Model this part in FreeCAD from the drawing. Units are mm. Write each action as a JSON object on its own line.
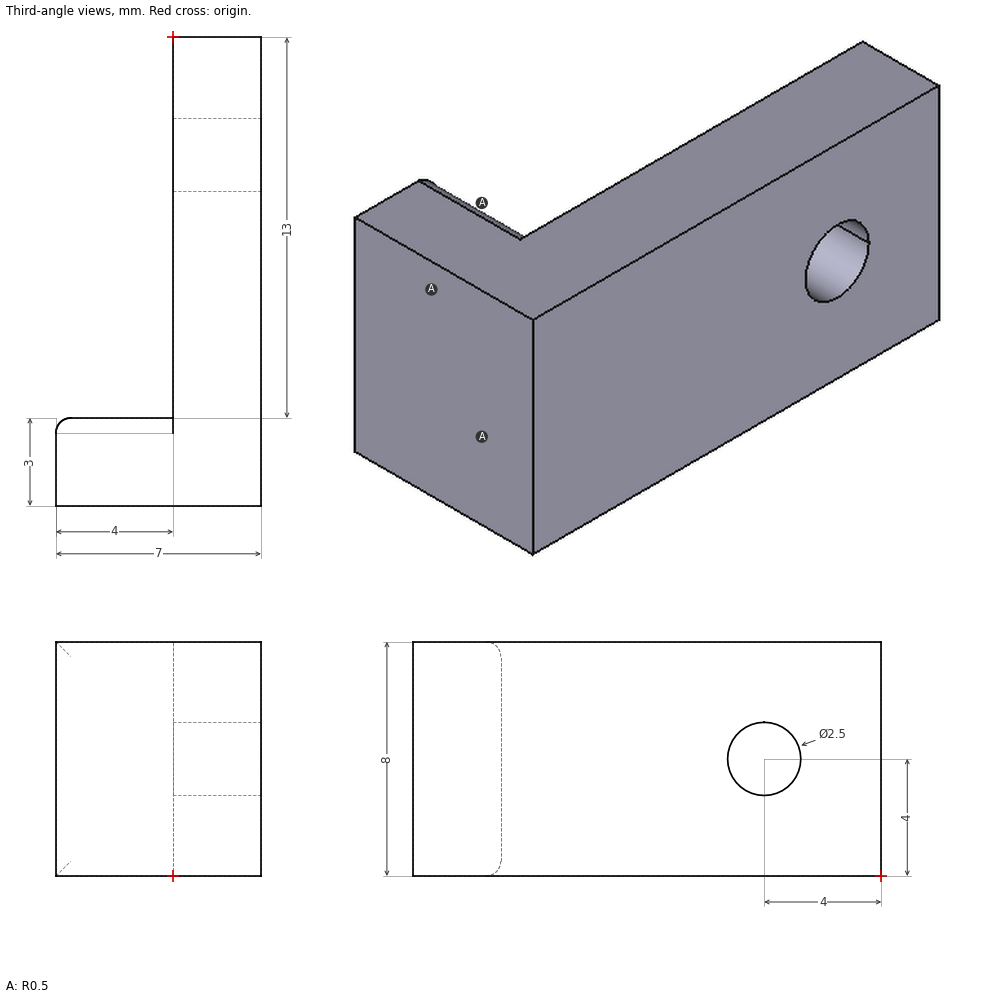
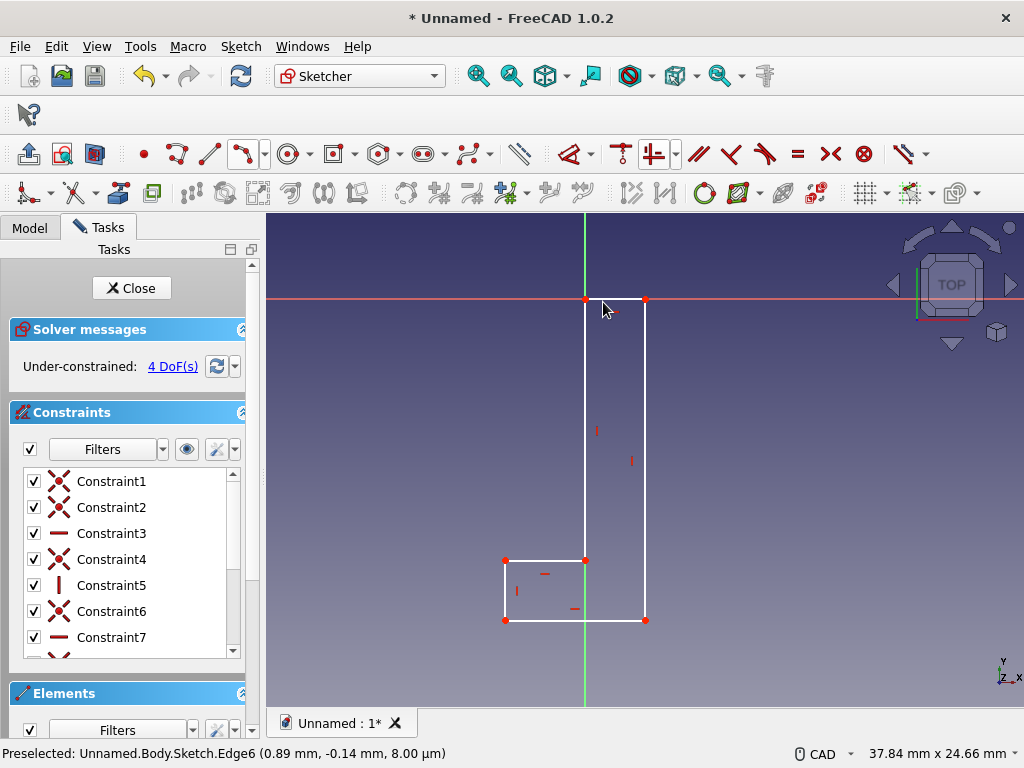
{"action": "left_click", "coordinate": [568, 154]}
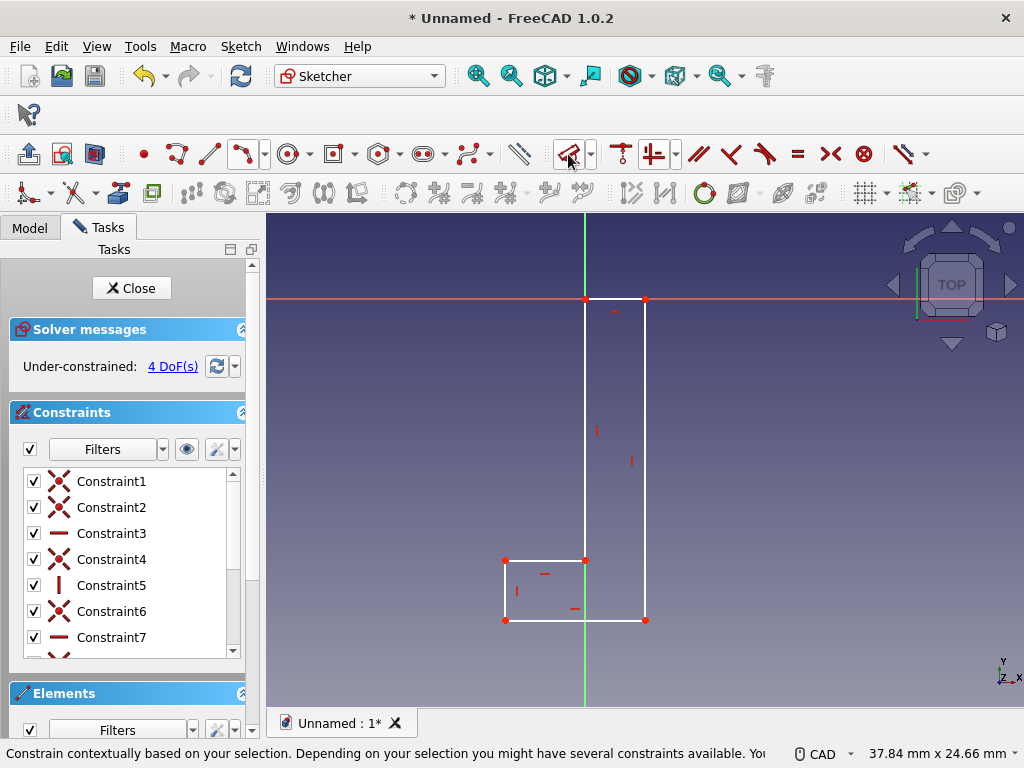
{"action": "left_click", "coordinate": [561, 561]}
{"action": "left_click", "coordinate": [545, 595]}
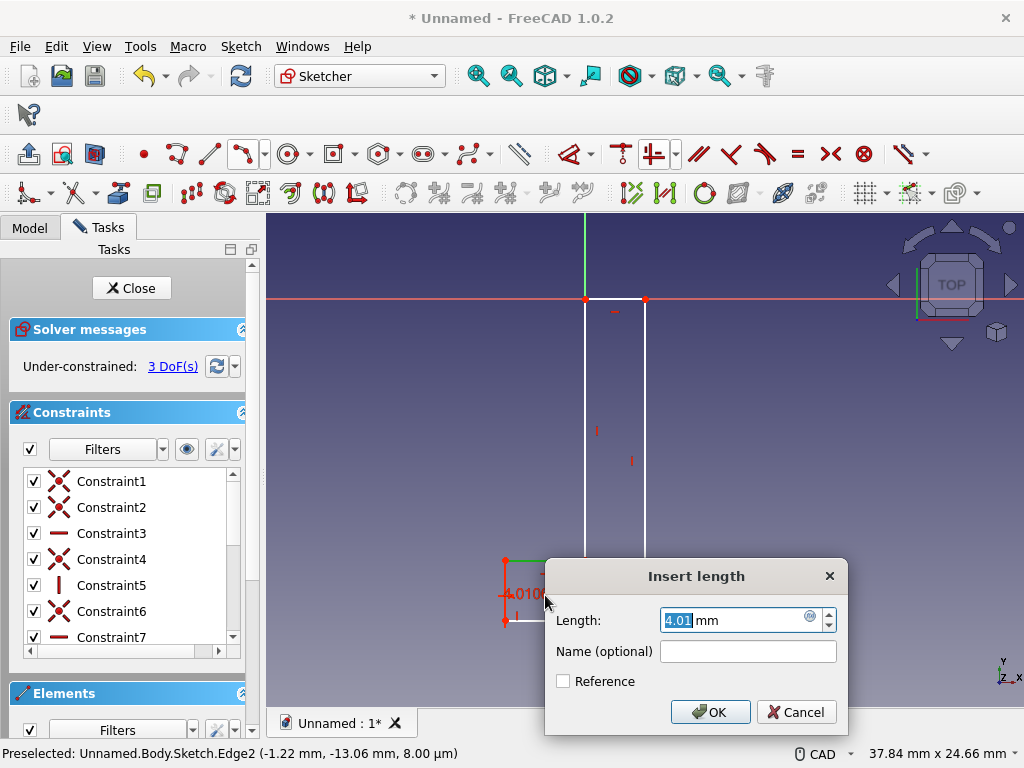
{"action": "type", "text": "4"}
{"action": "key", "text": "Return"}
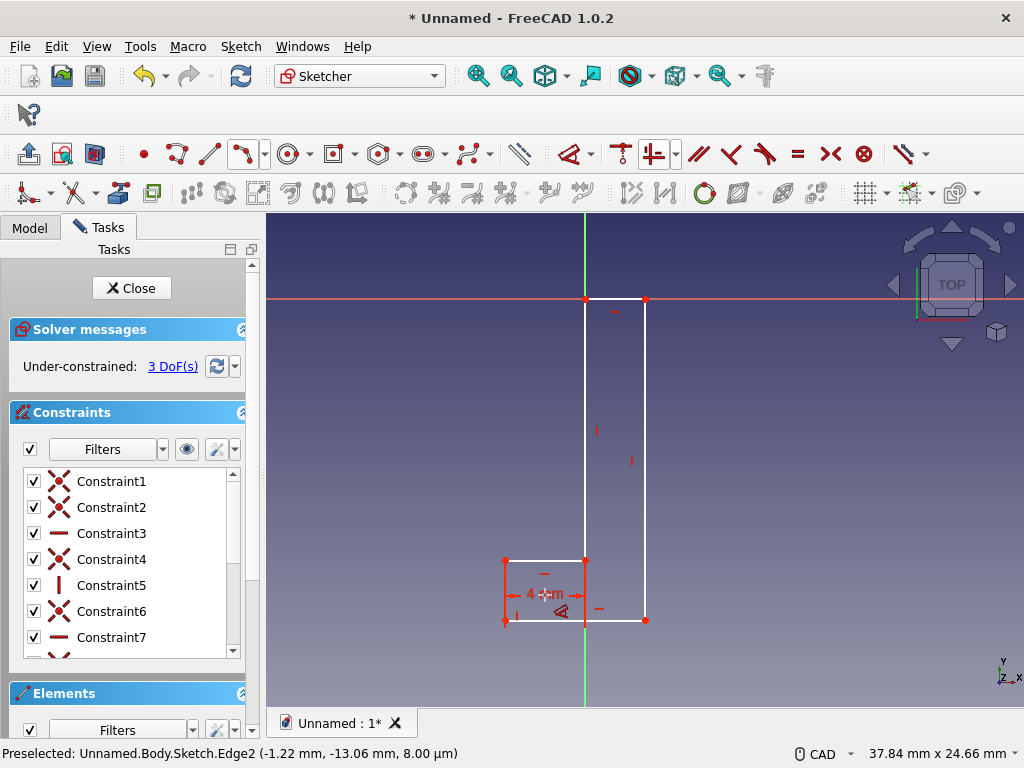
{"action": "left_click", "coordinate": [505, 579]}
{"action": "left_click", "coordinate": [471, 591]}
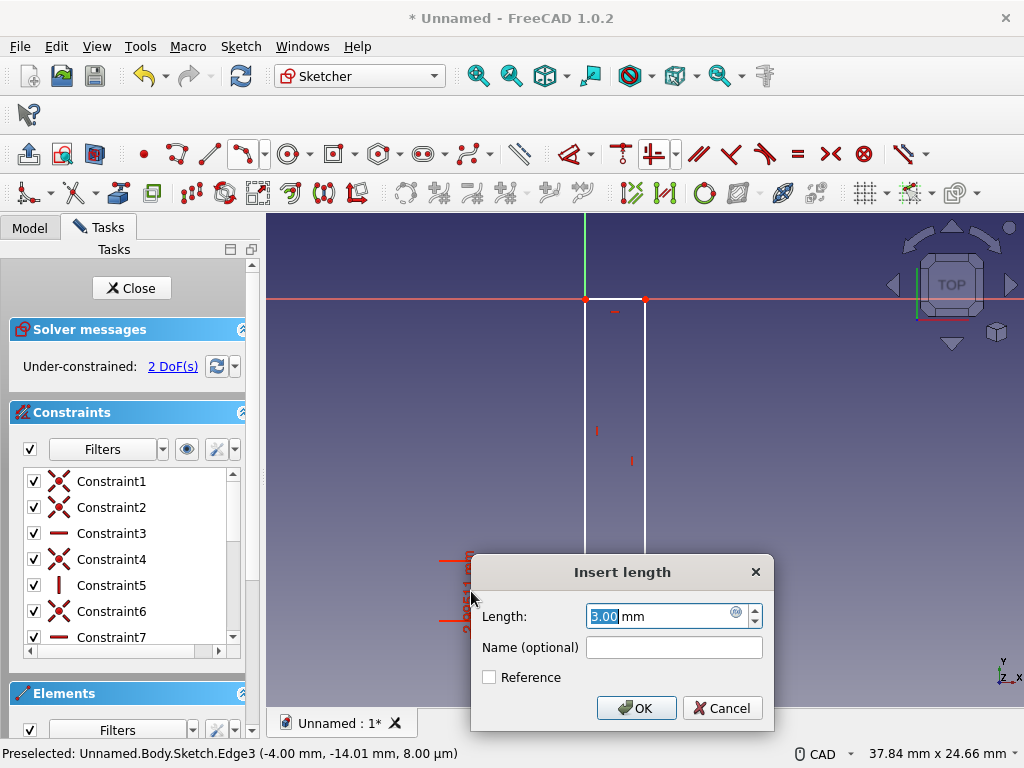
{"action": "type", "text": "3"}
{"action": "key", "text": "Return"}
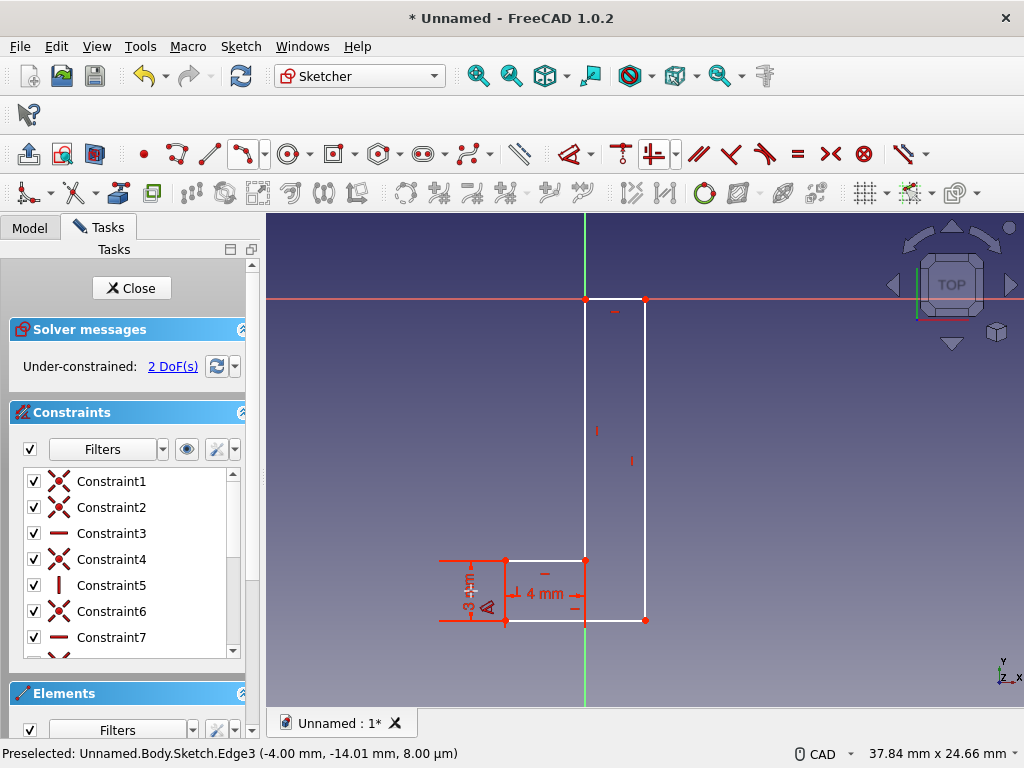
{"action": "left_click", "coordinate": [547, 621]}
{"action": "left_click", "coordinate": [543, 655]}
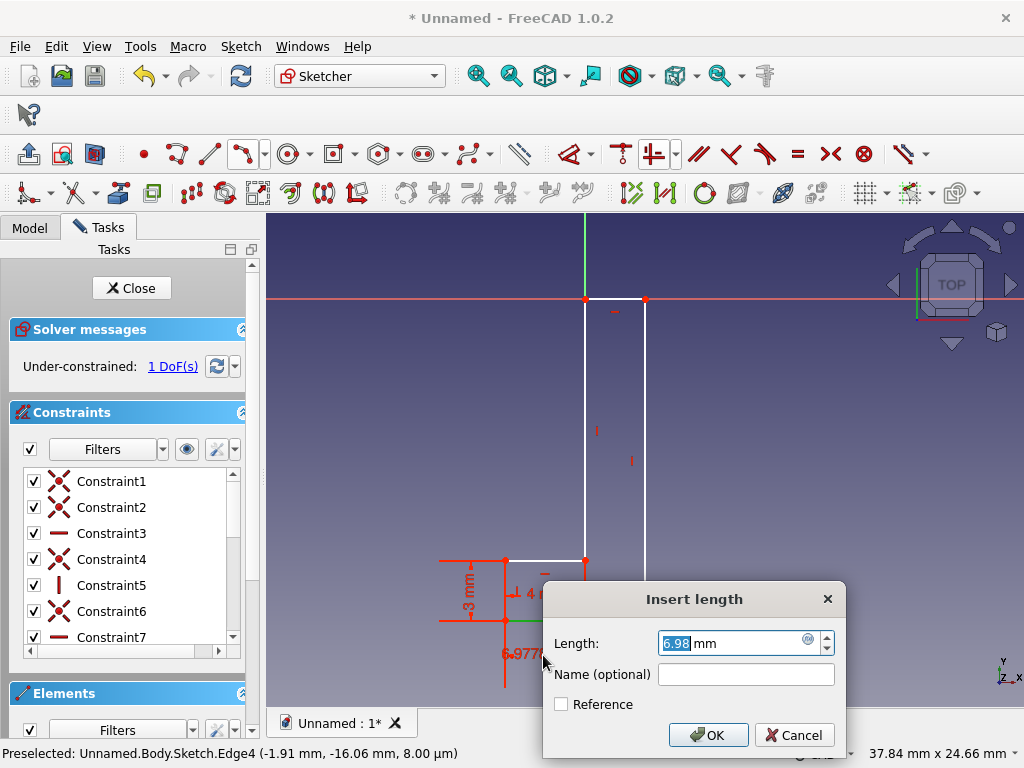
{"action": "type", "text": "7"}
{"action": "key", "text": "Return"}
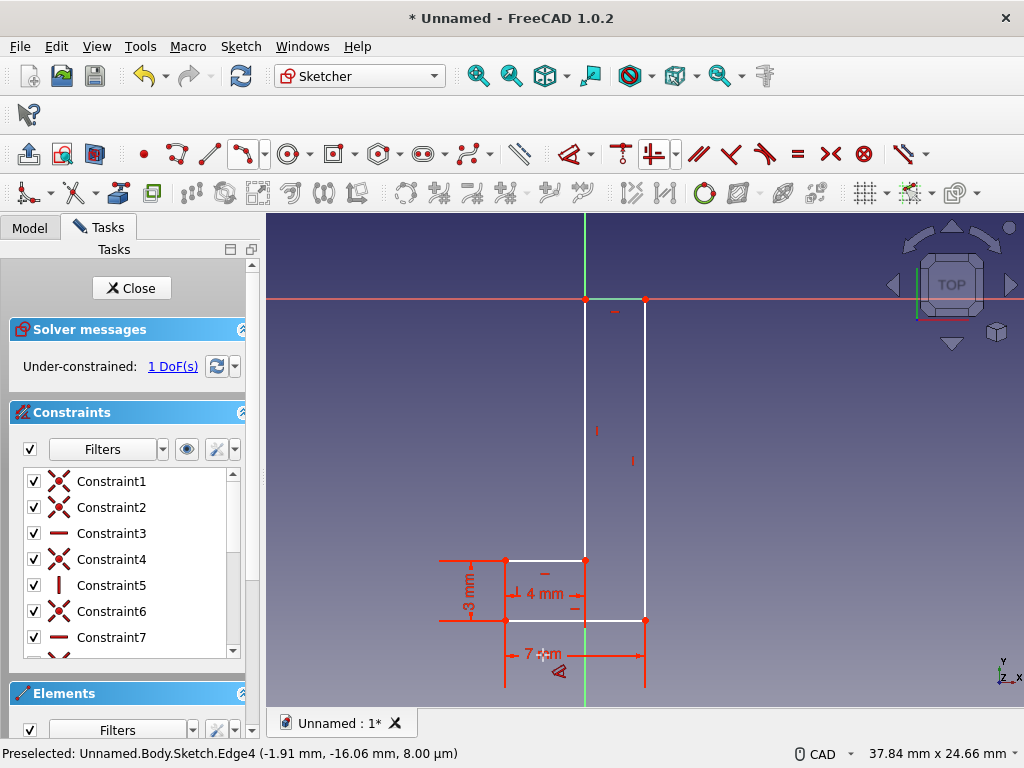
{"action": "left_click", "coordinate": [585, 378]}
{"action": "left_click", "coordinate": [619, 430]}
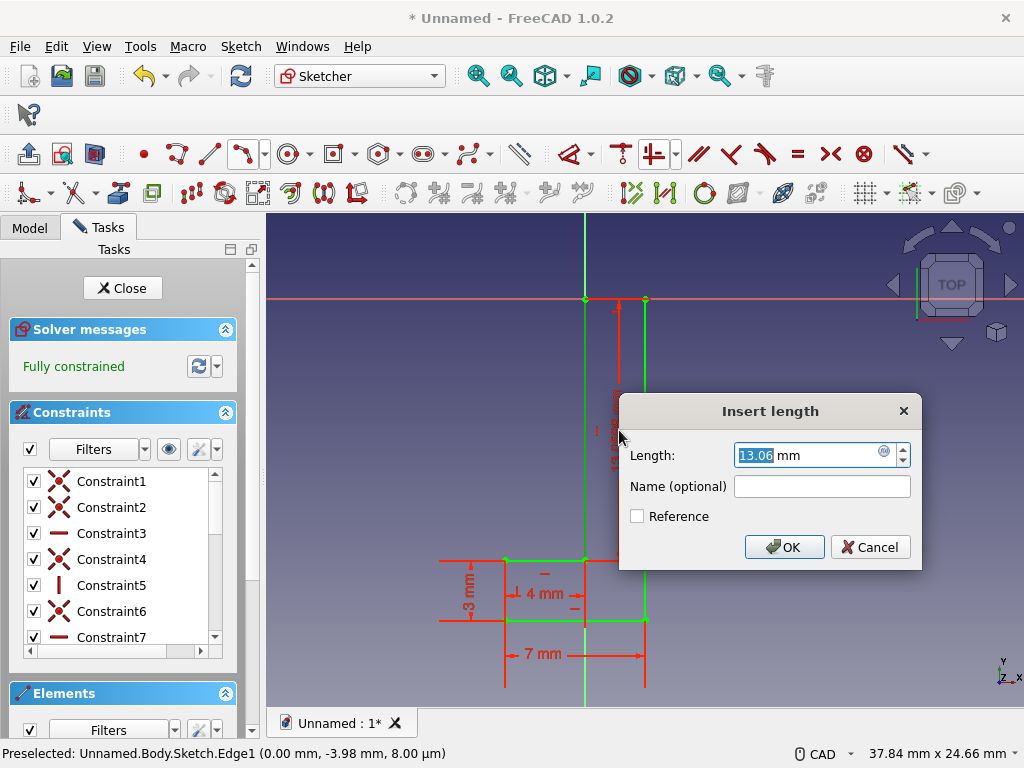
{"action": "type", "text": "13"}
{"action": "key", "text": "Return"}
{"action": "key", "text": "Escape"}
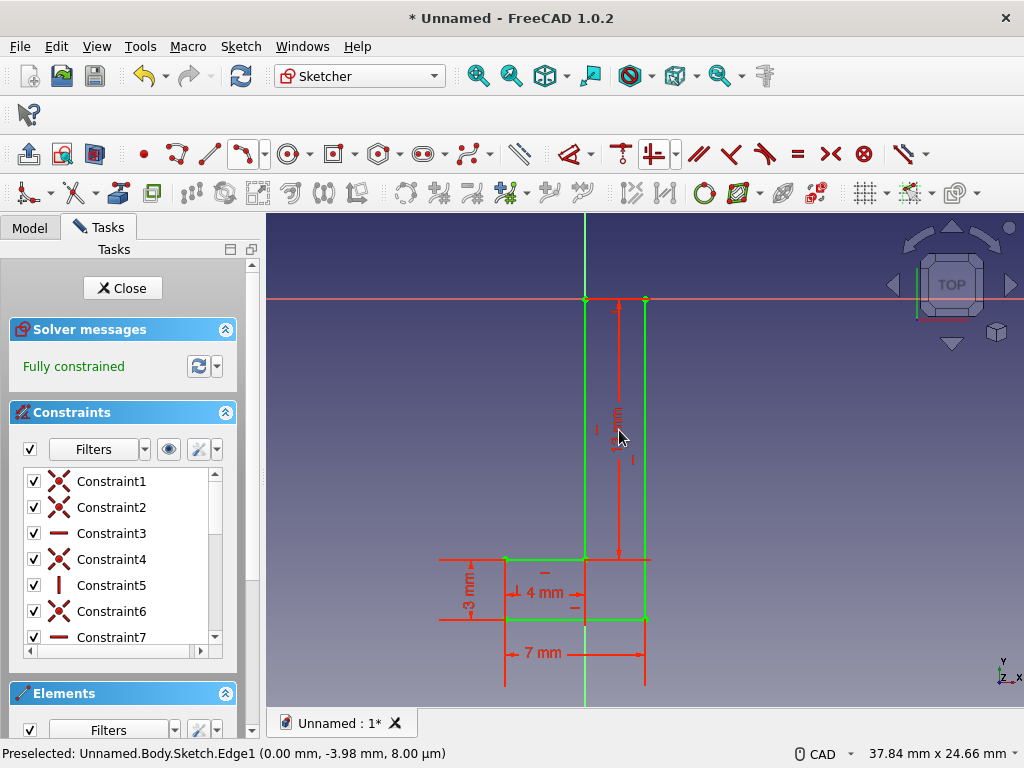
{"action": "left_click", "coordinate": [123, 288]}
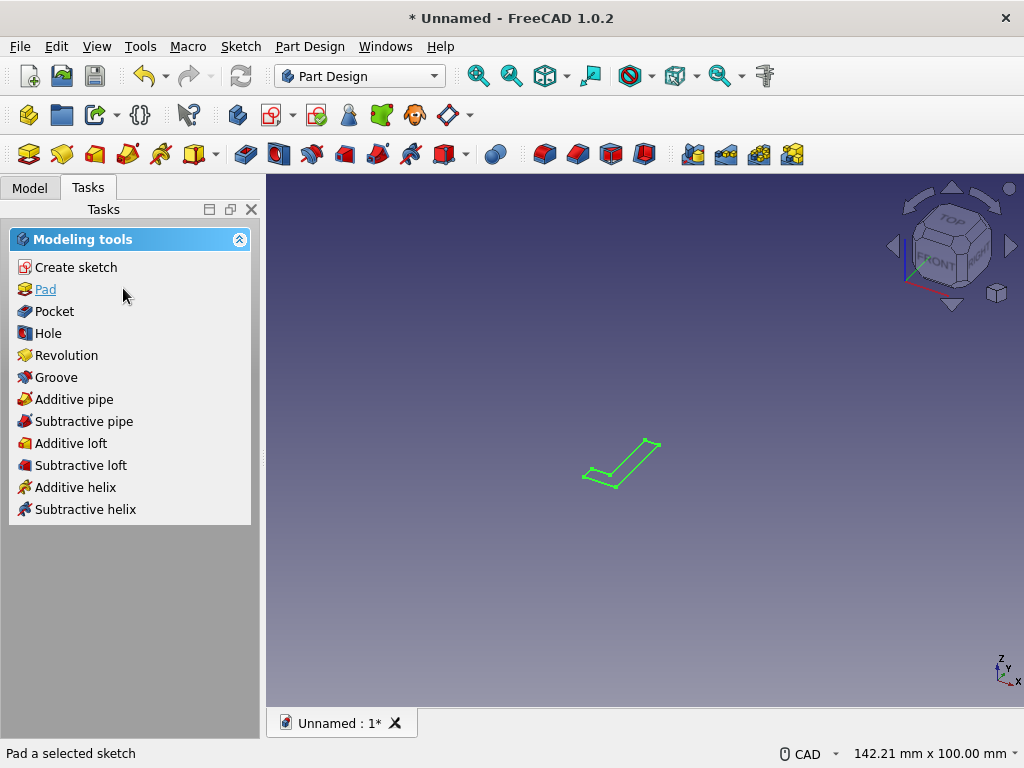
{"action": "left_click", "coordinate": [29, 154]}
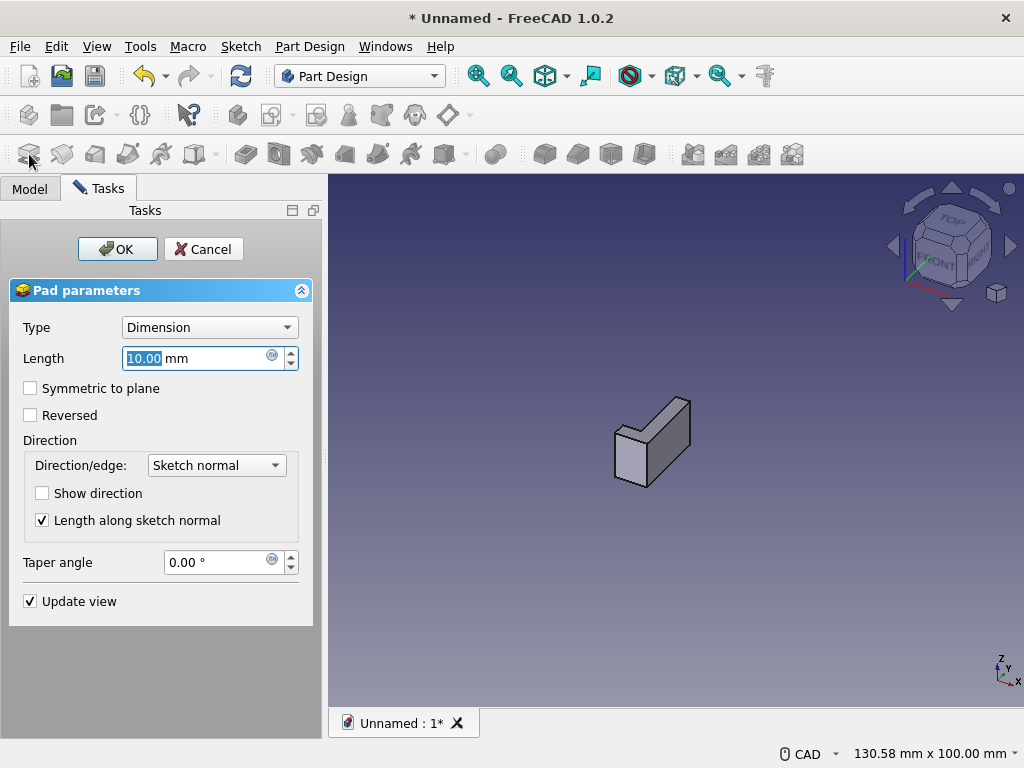
{"action": "type", "text": "8"}
{"action": "key", "text": "Tab"}